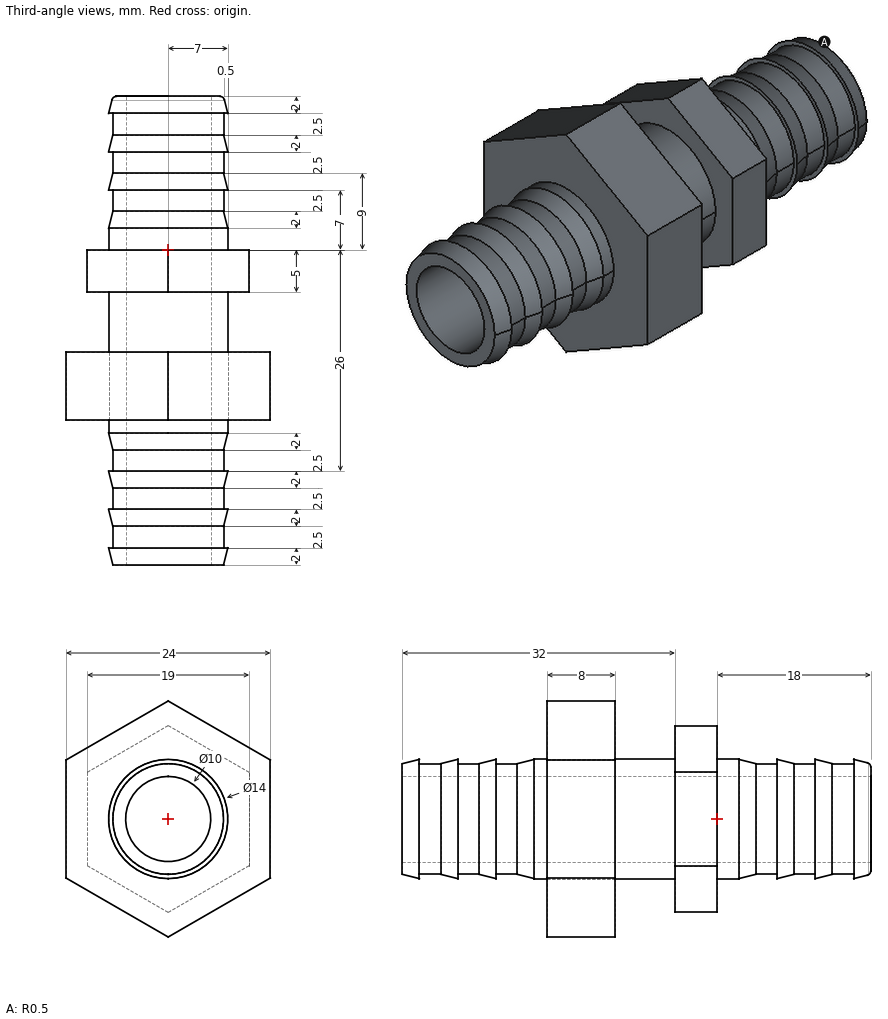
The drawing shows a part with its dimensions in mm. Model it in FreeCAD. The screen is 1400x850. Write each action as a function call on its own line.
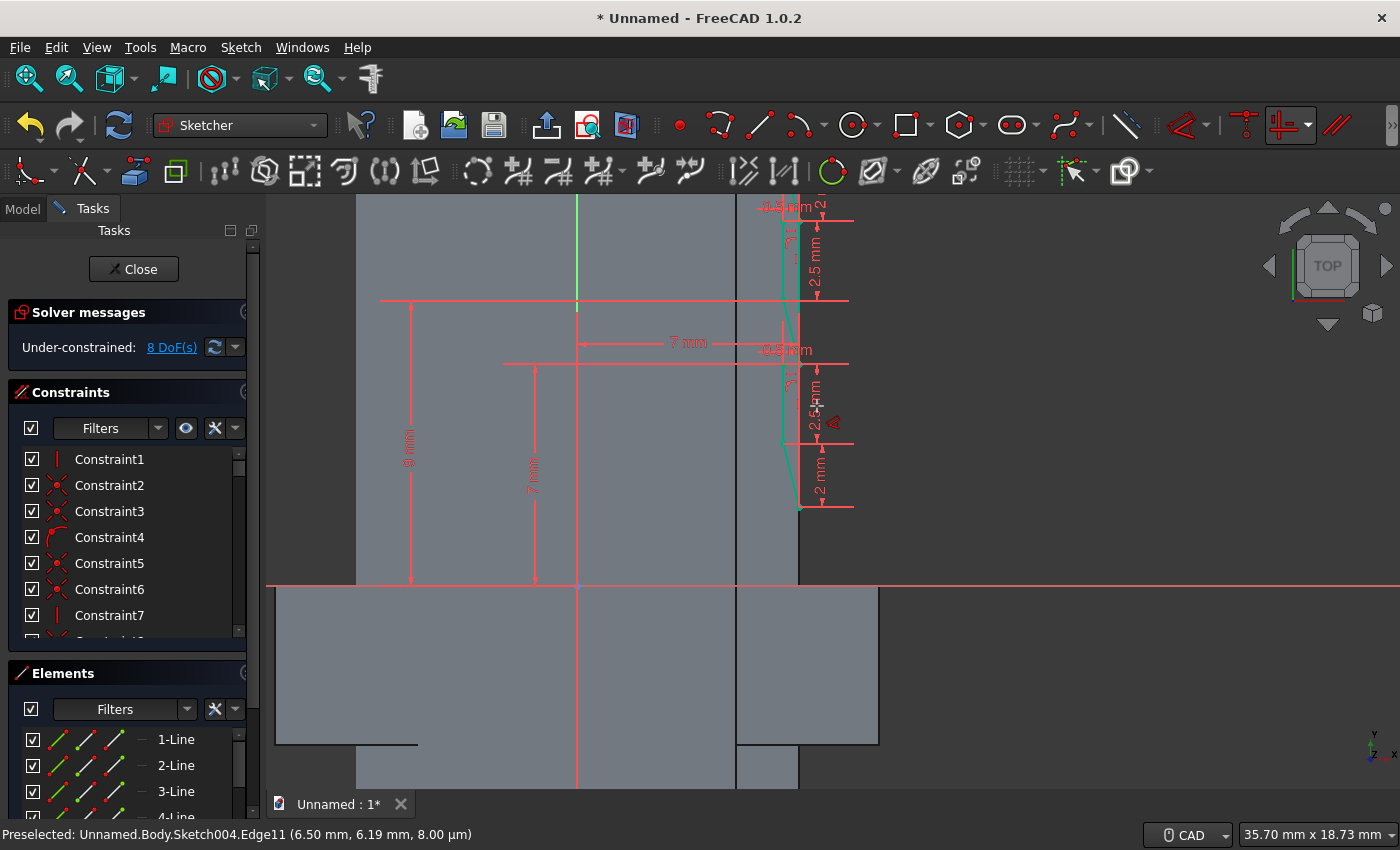
scroll(784, 391, down, 8)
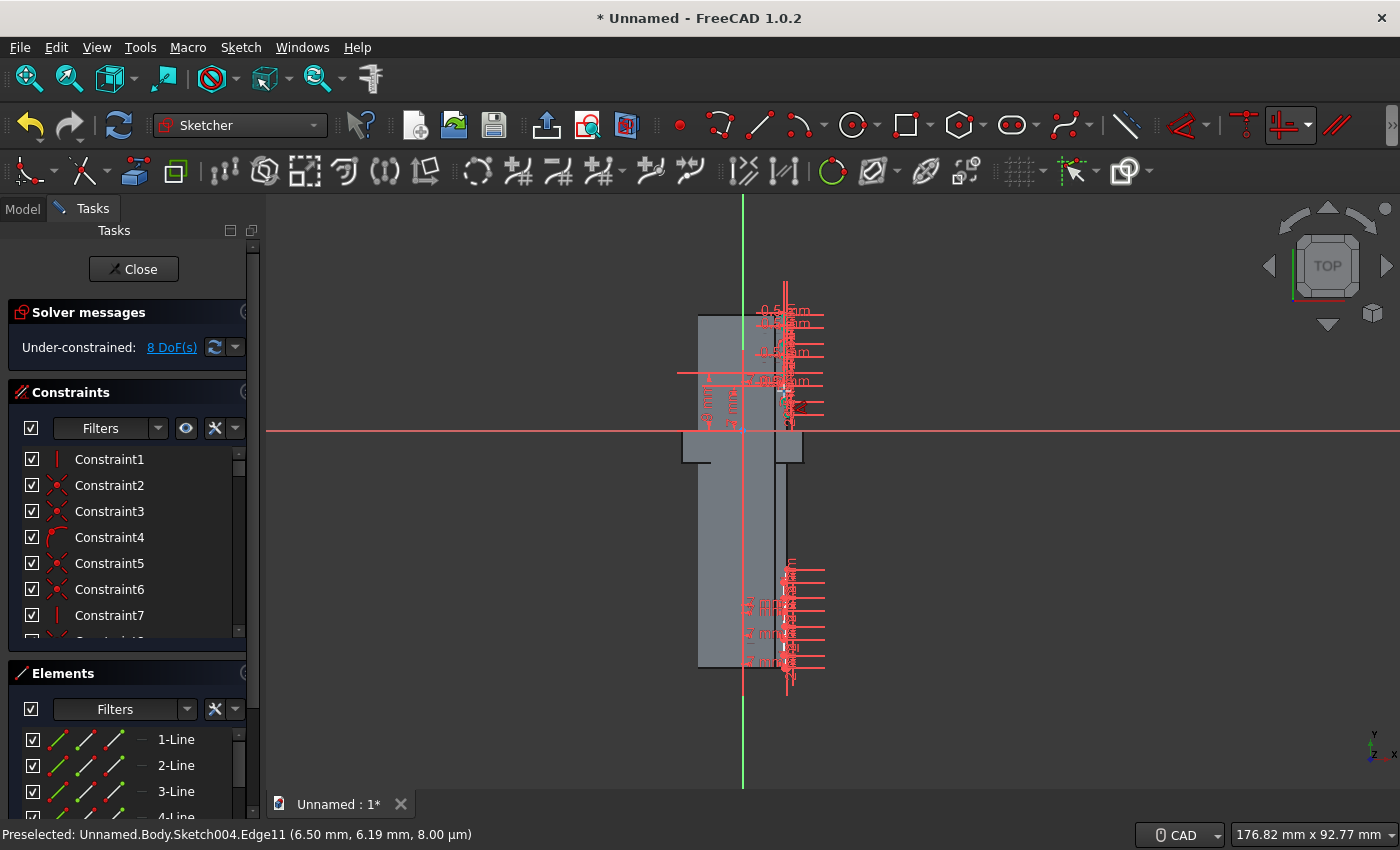
scroll(784, 587, up, 7)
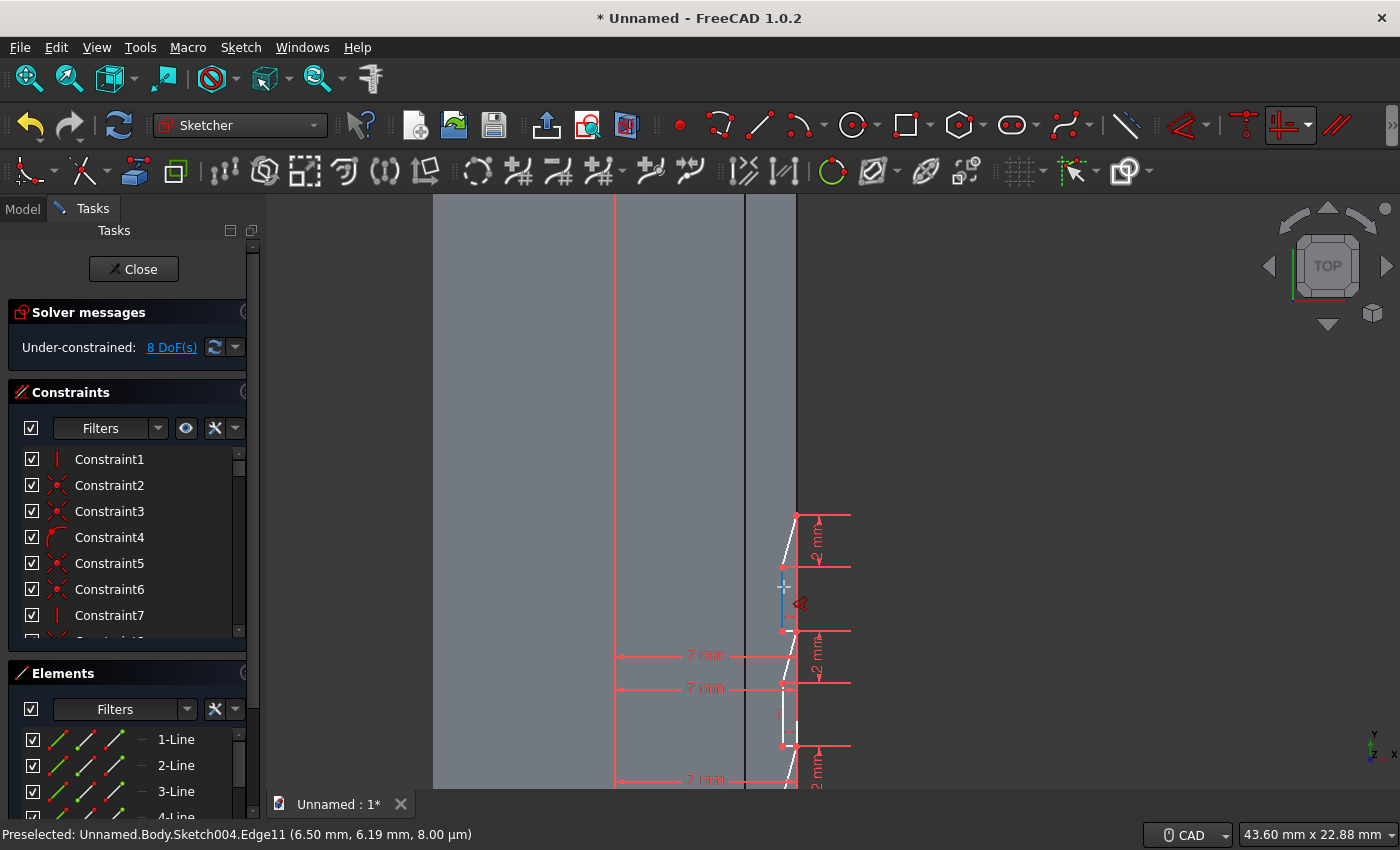
click(782, 586)
click(816, 599)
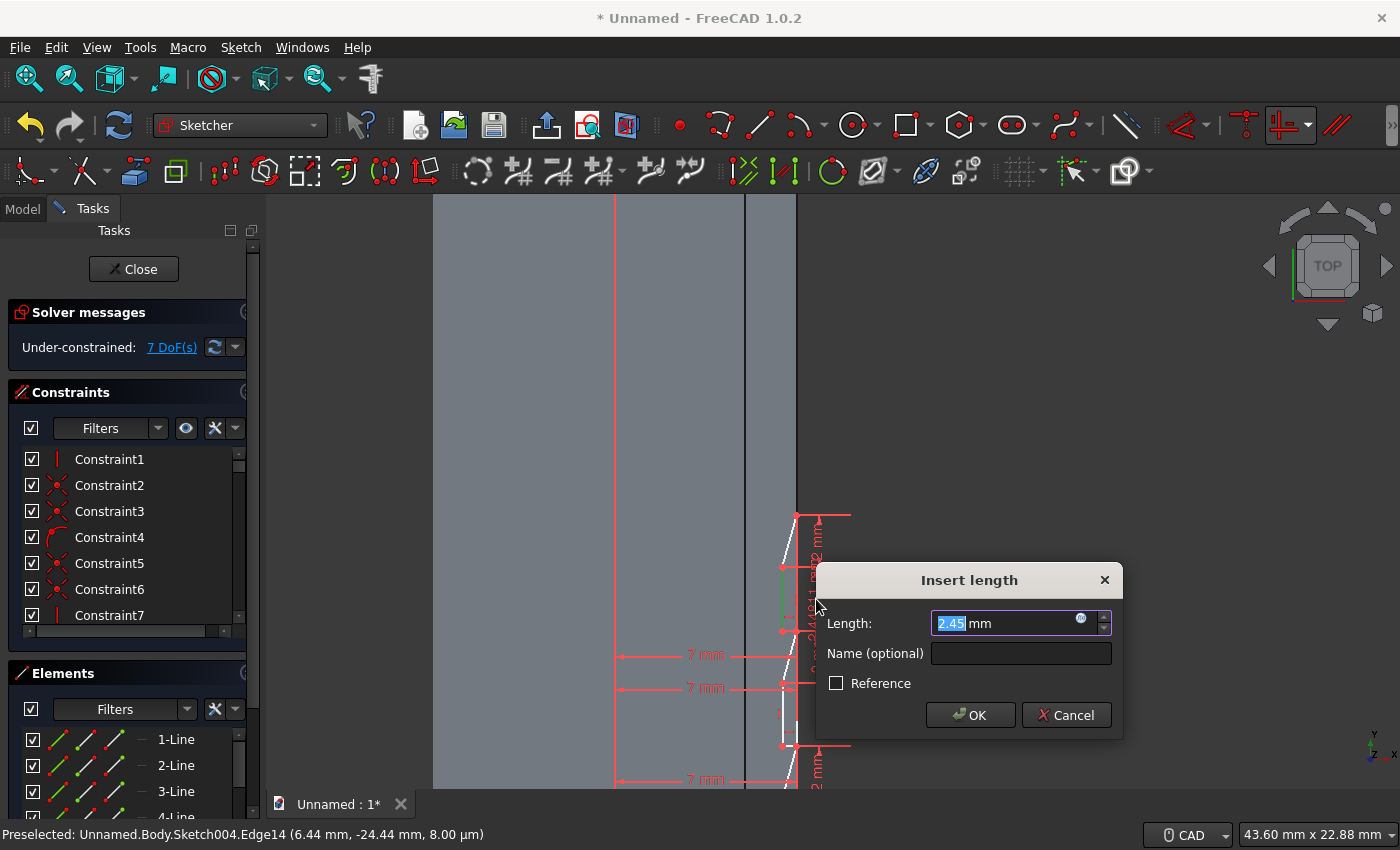
text(2.5)
key(Return)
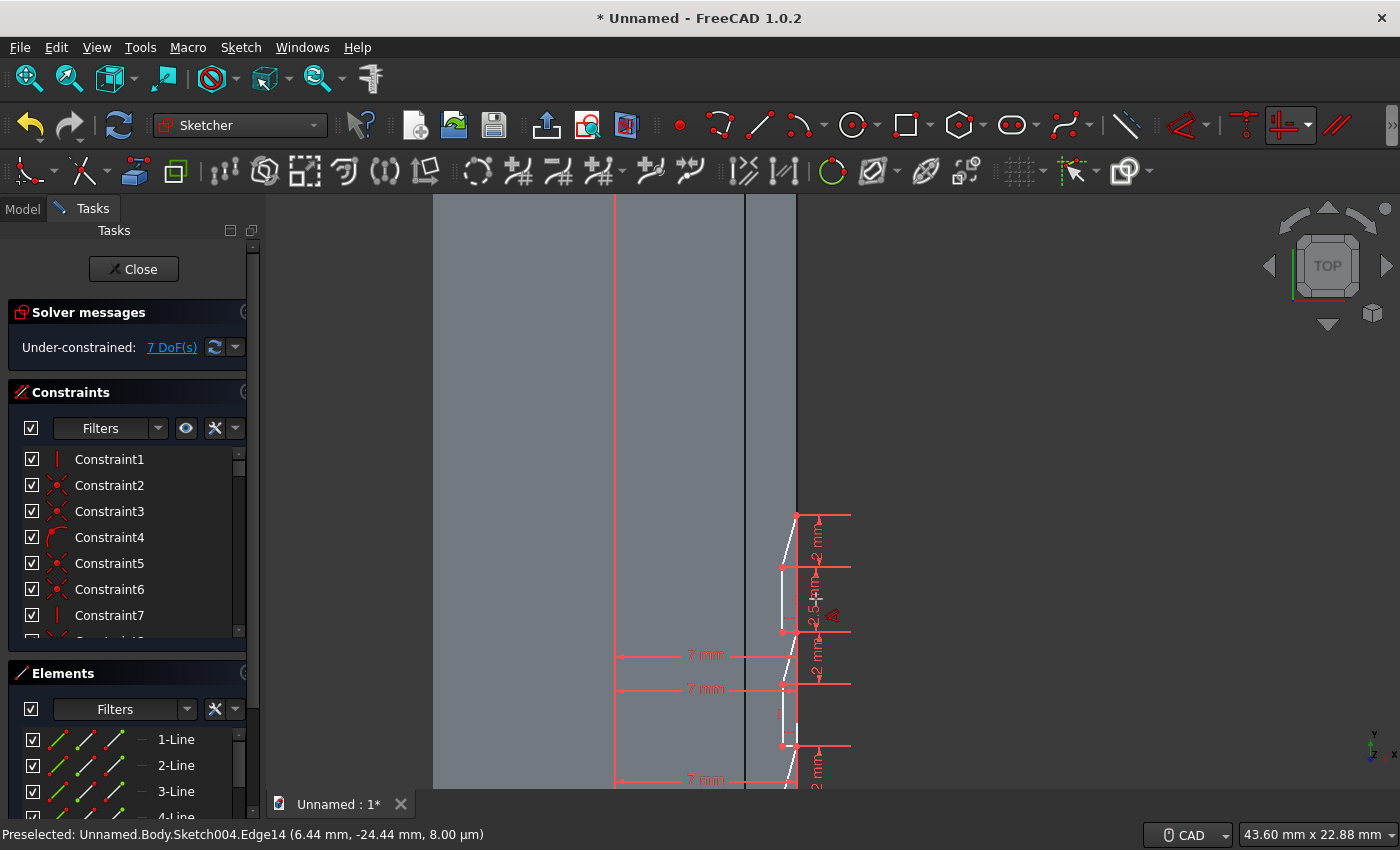
scroll(789, 632, up, 6)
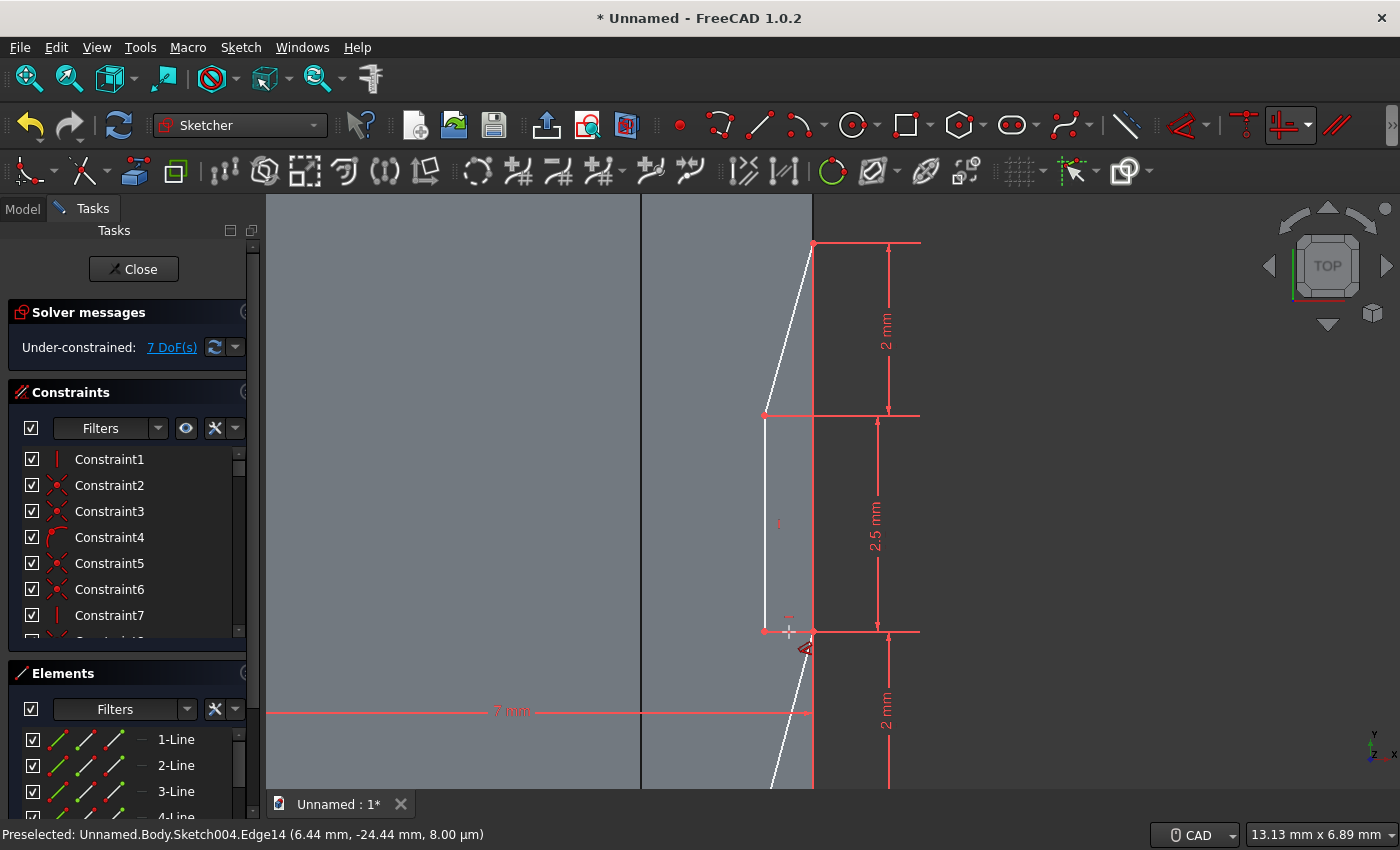
click(789, 632)
click(789, 666)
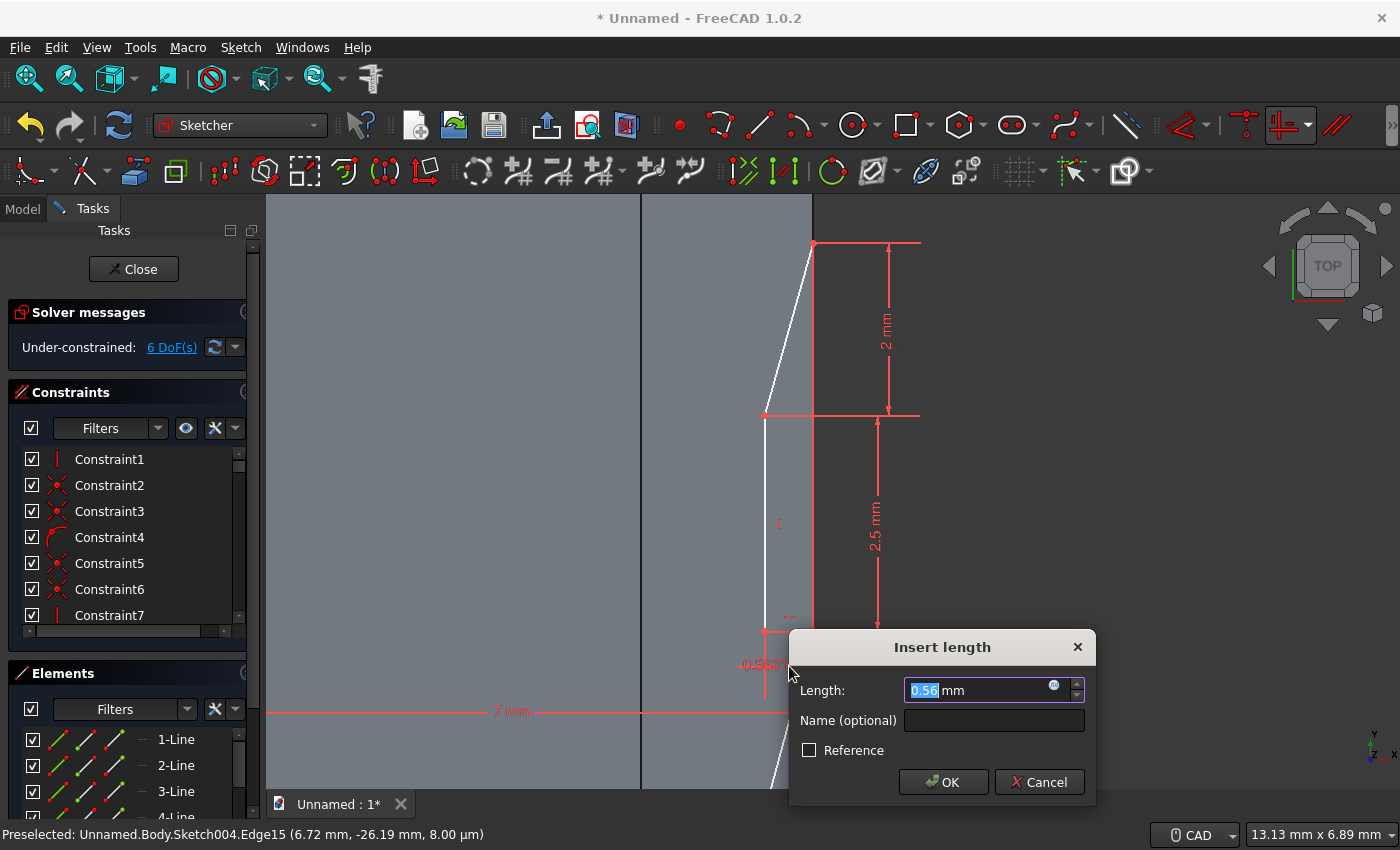
text(0.5)
key(Return)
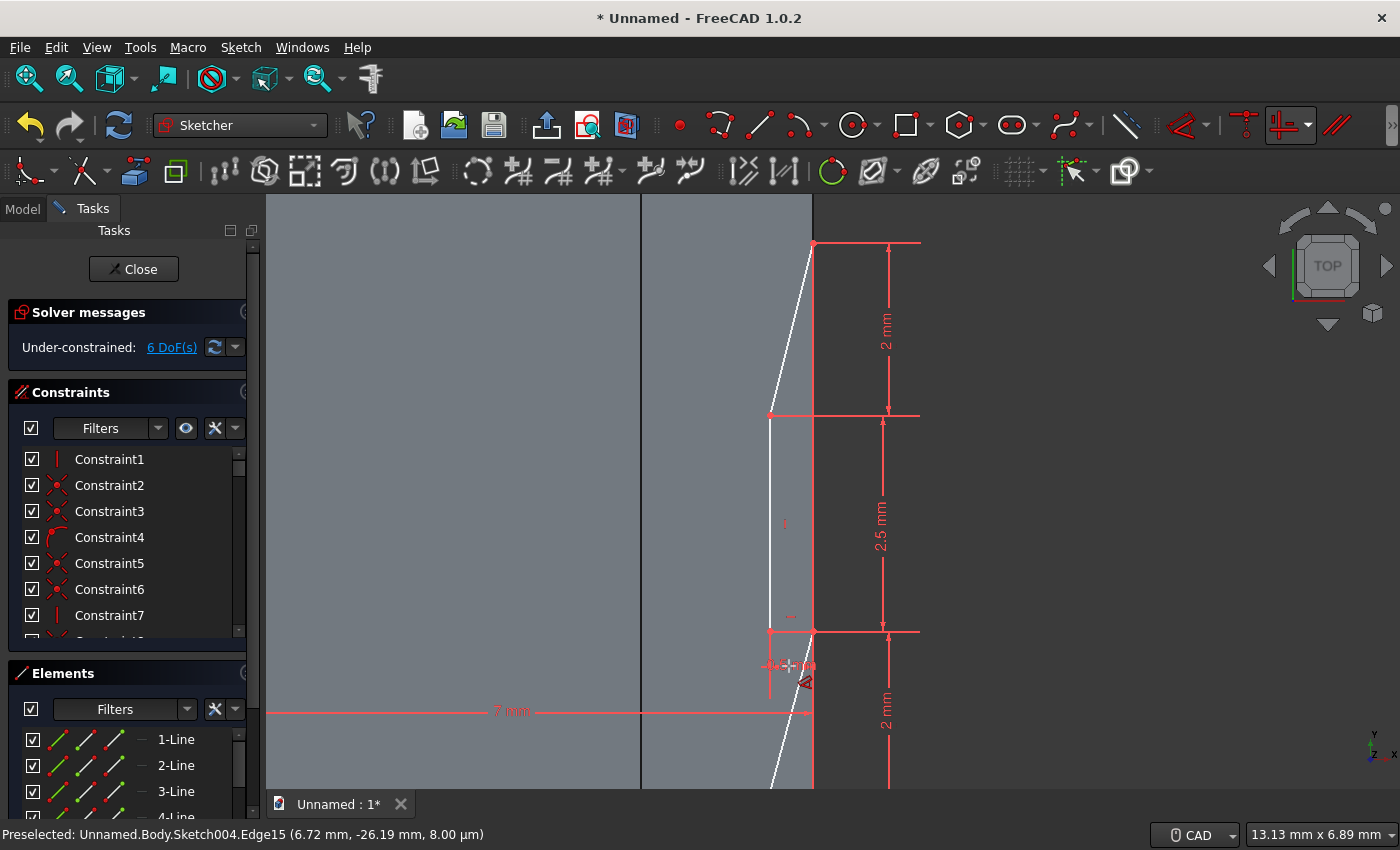
scroll(785, 596, down, 13)